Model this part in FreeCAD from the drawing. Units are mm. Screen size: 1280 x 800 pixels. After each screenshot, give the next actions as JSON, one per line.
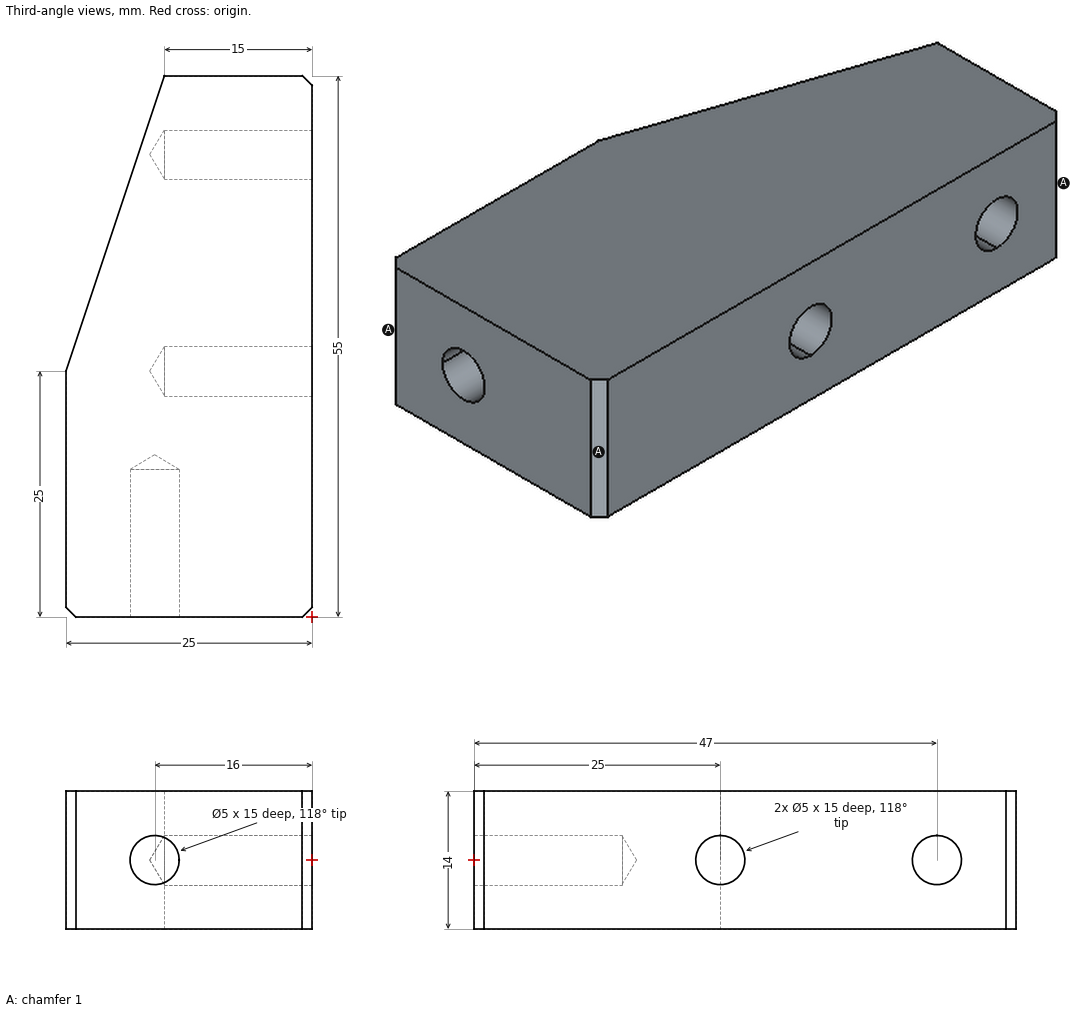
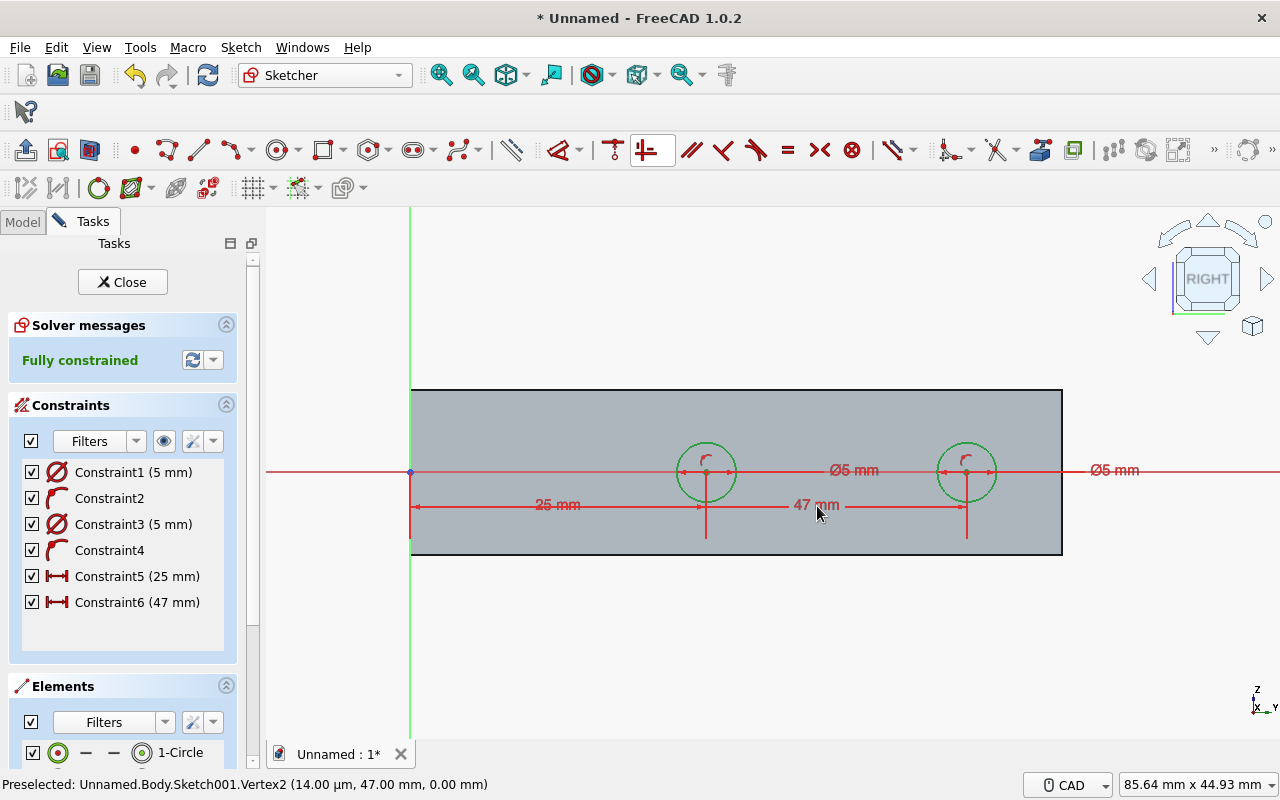
{"action": "left_click", "coordinate": [123, 282]}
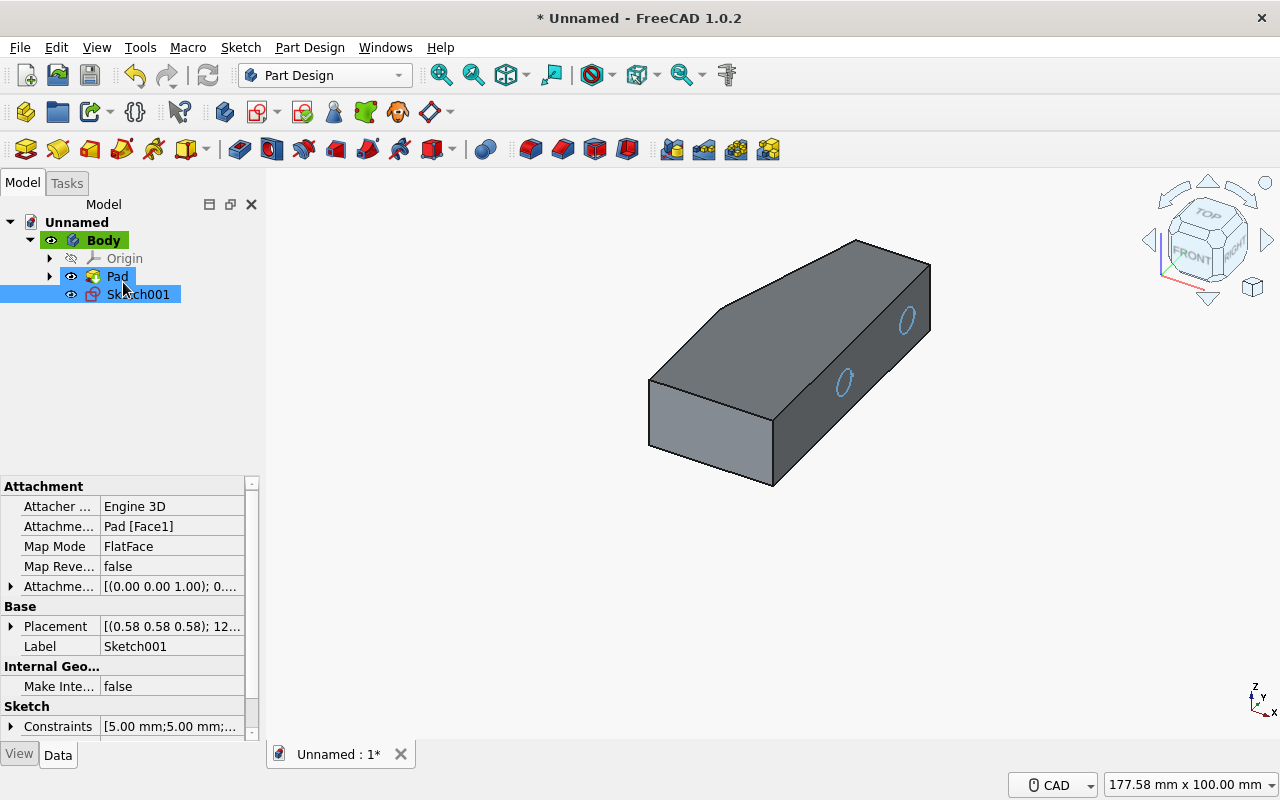
{"action": "left_click", "coordinate": [272, 150]}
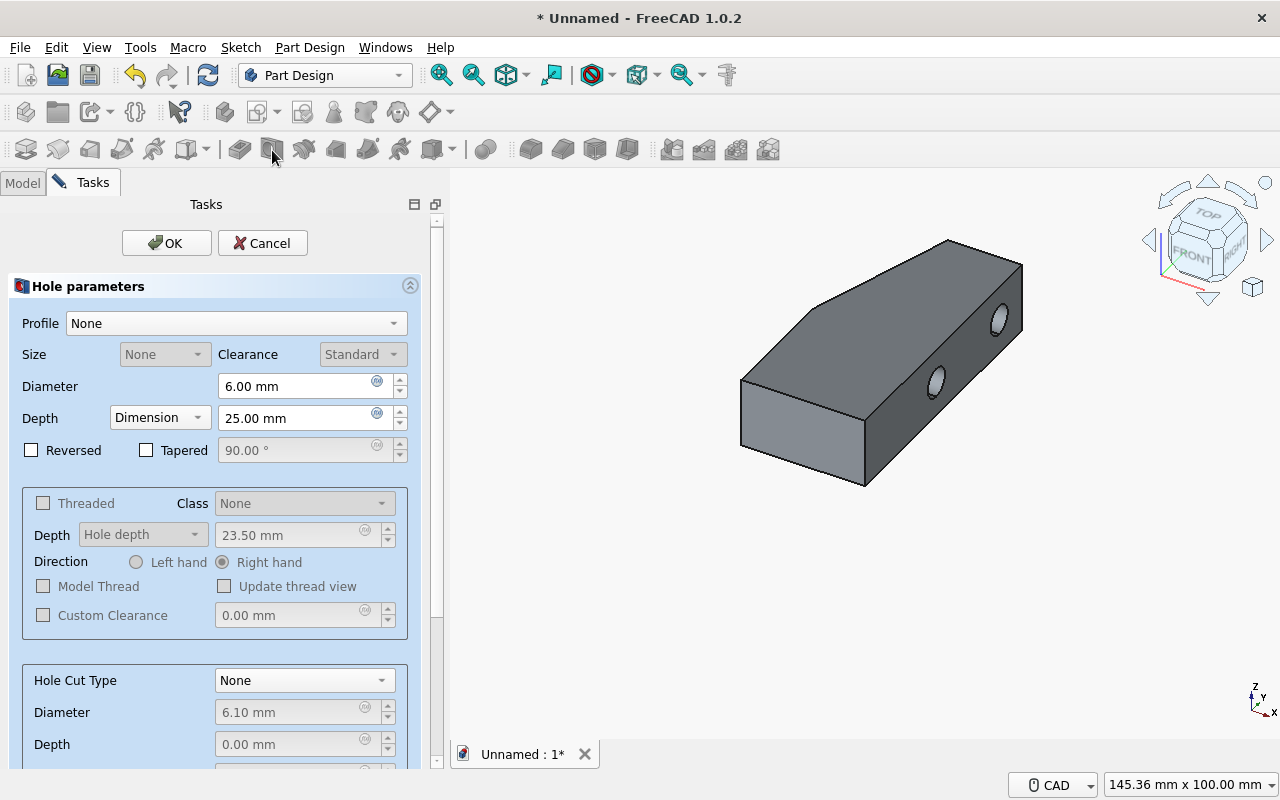
{"action": "triple_click", "coordinate": [305, 386]}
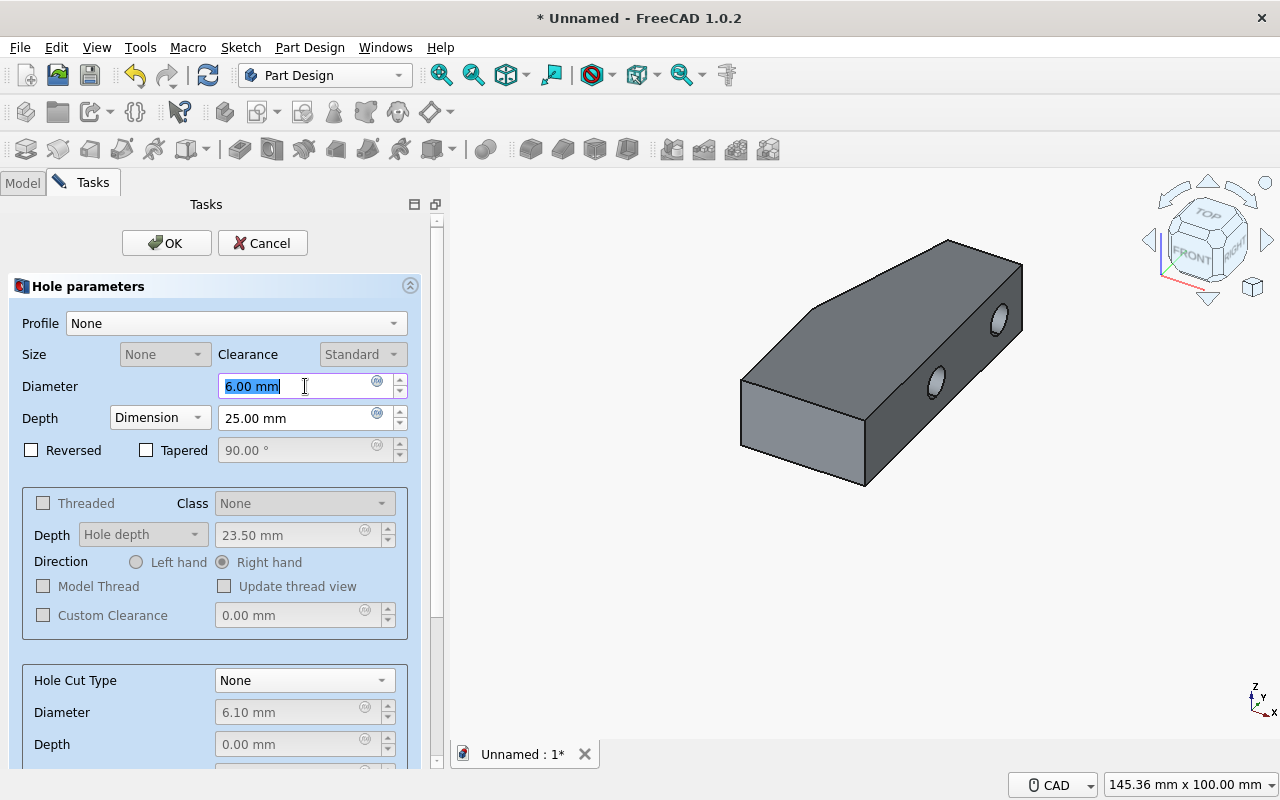
{"action": "type", "text": "5"}
{"action": "key", "text": "Tab"}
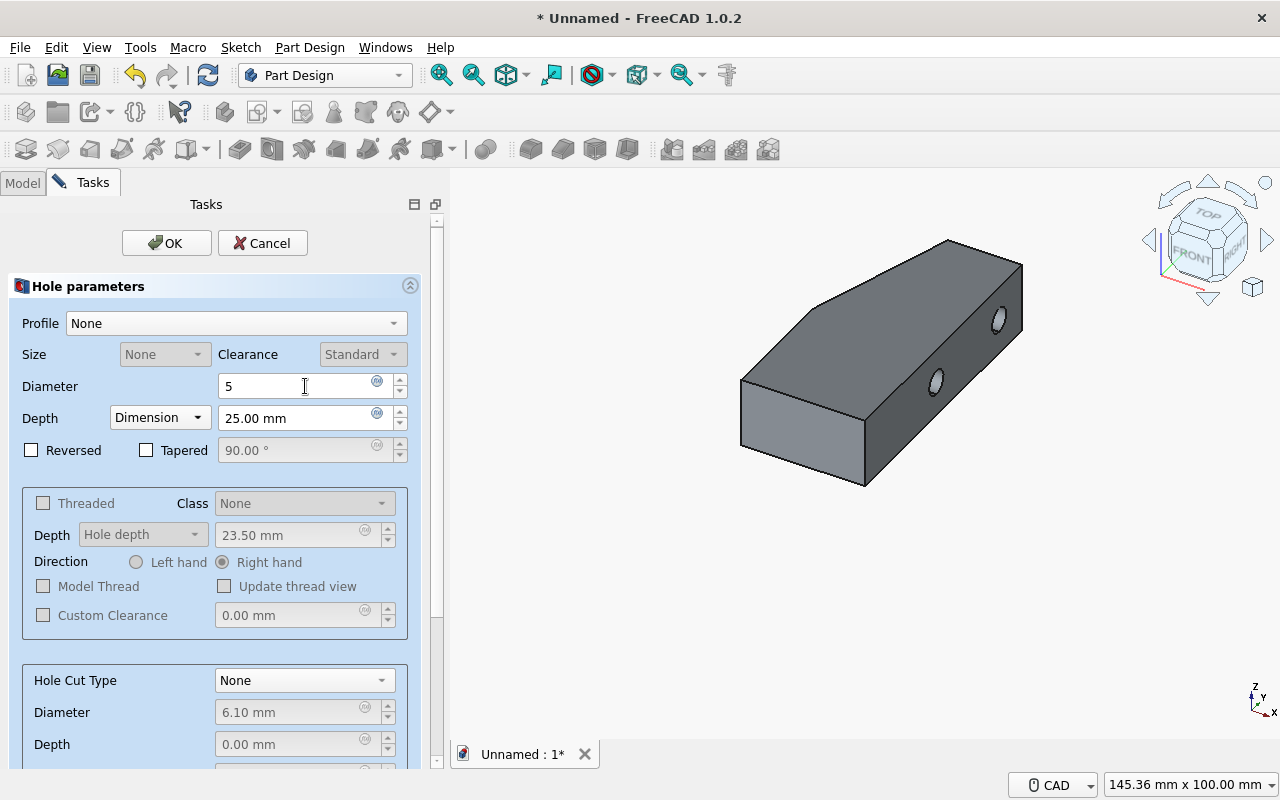
{"action": "triple_click", "coordinate": [305, 418]}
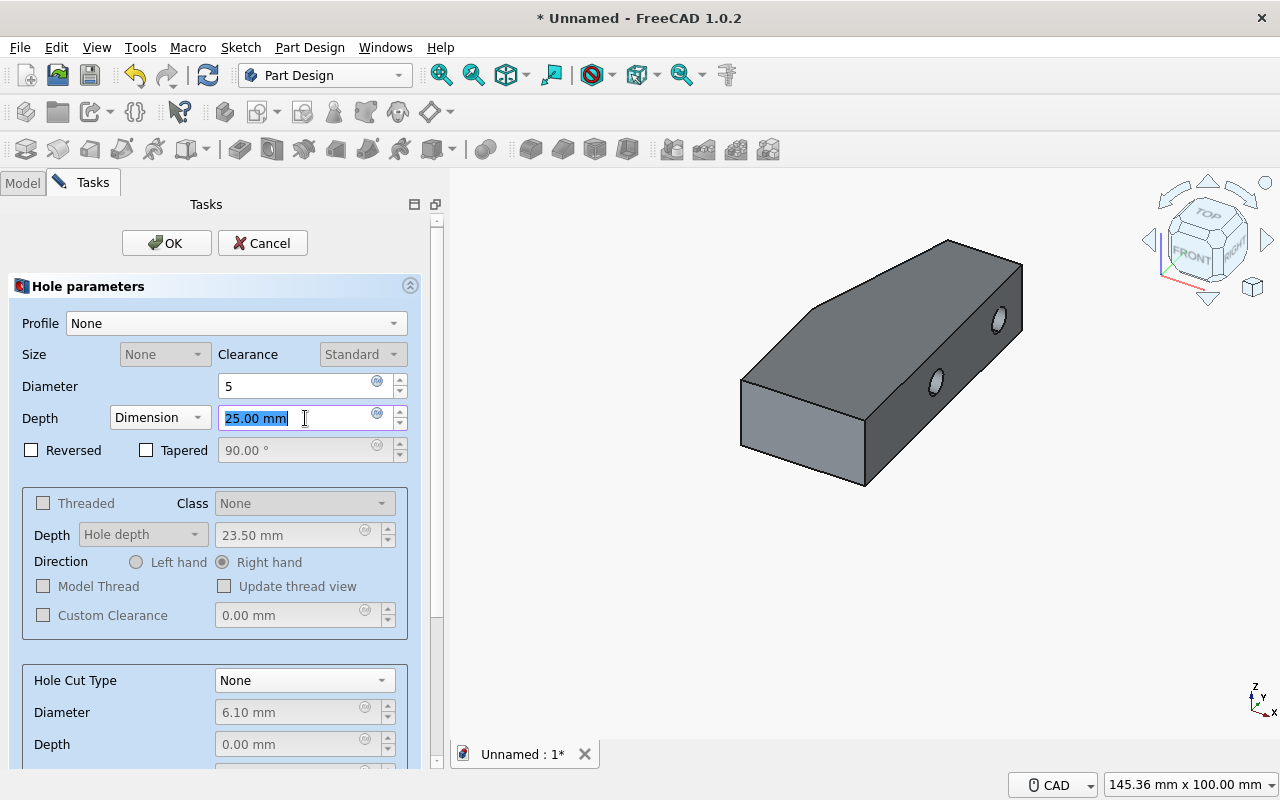
{"action": "type", "text": "15"}
{"action": "key", "text": "Tab"}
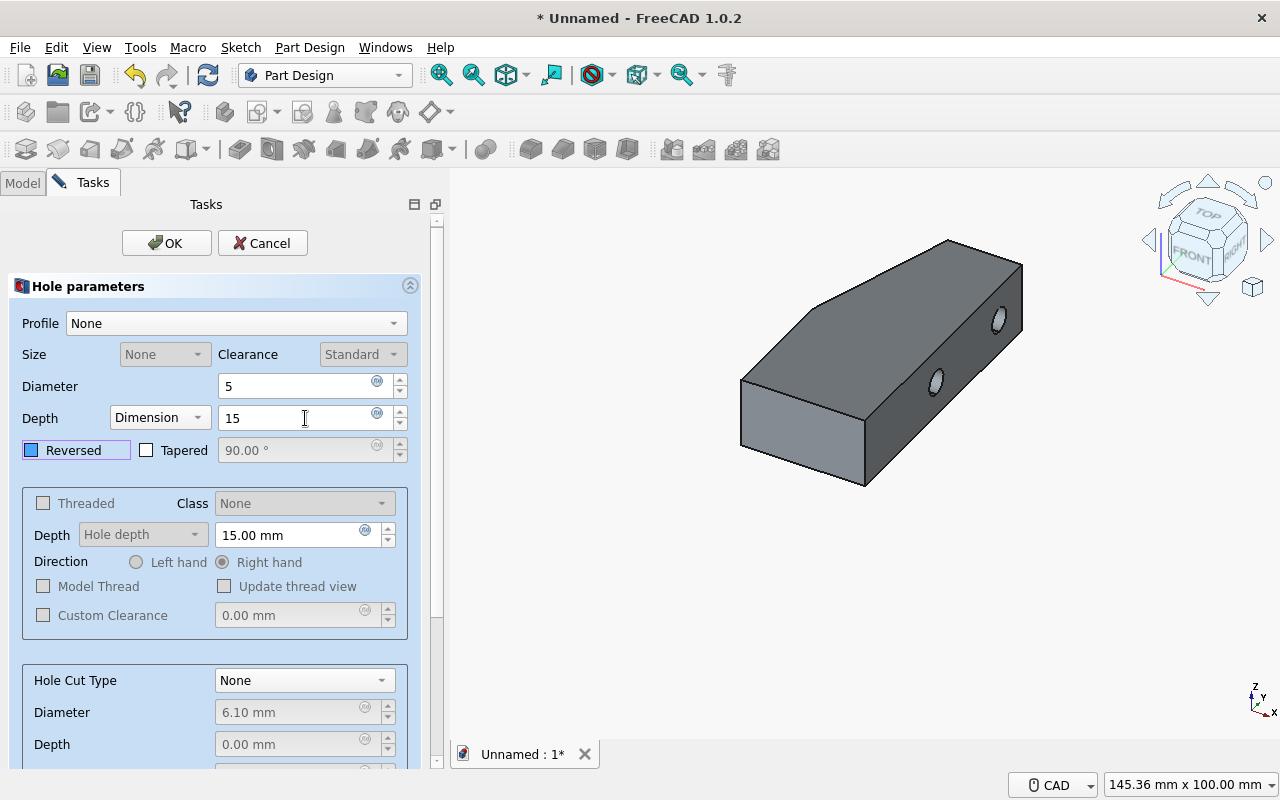
{"action": "left_click", "coordinate": [167, 243]}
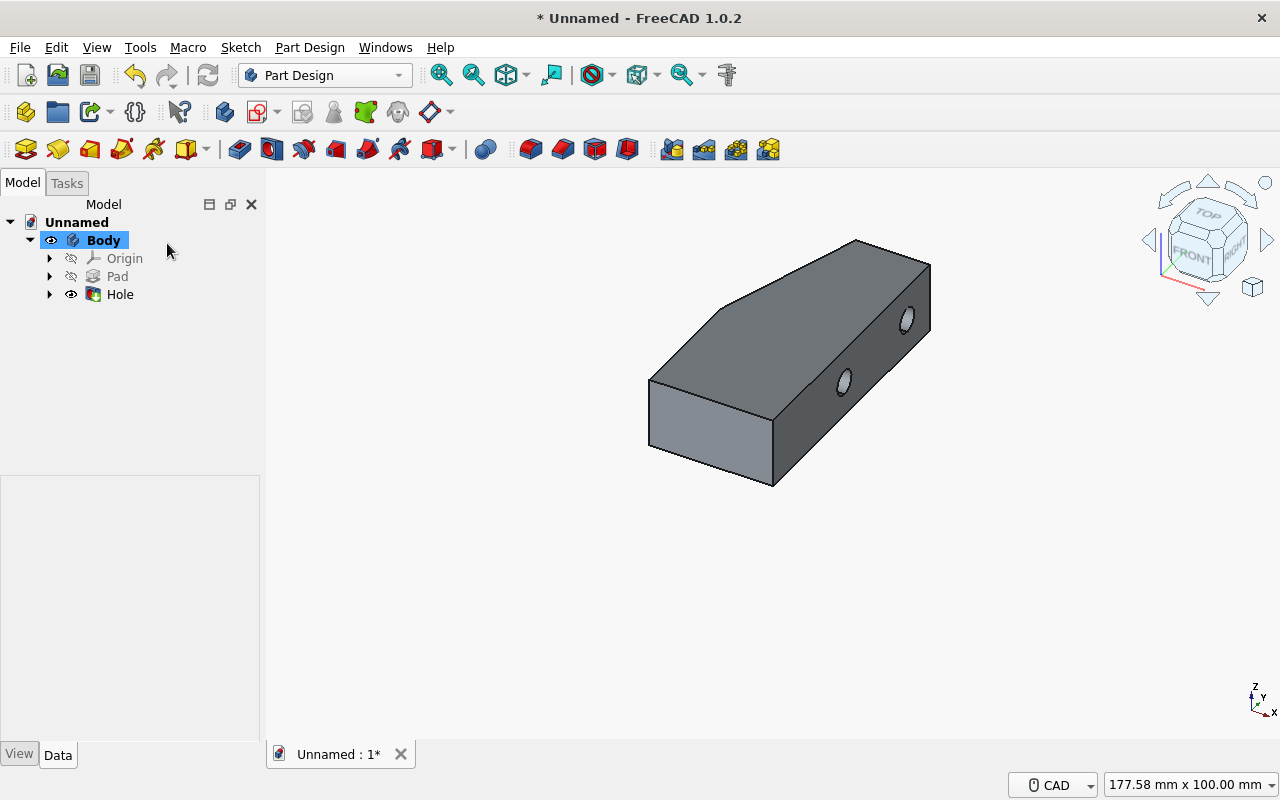
{"action": "left_click", "coordinate": [258, 112]}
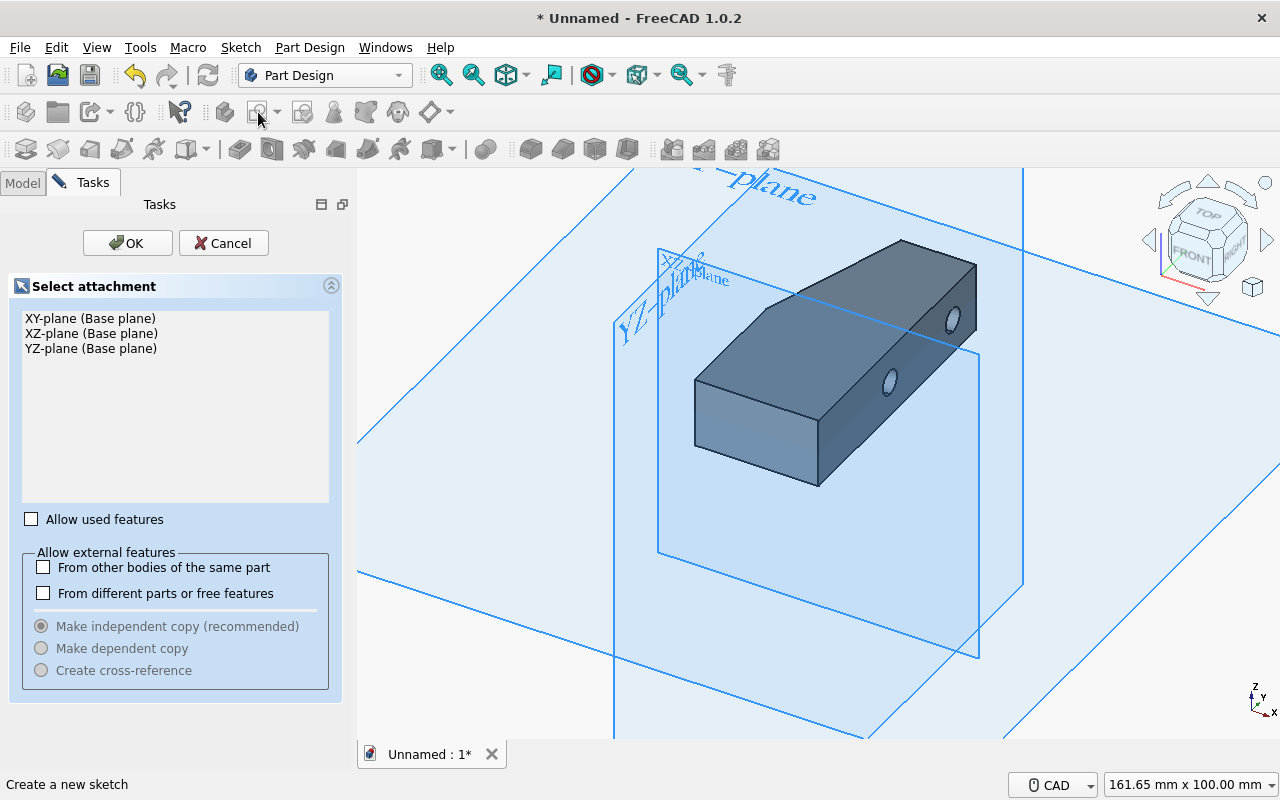
{"action": "left_click", "coordinate": [82, 334]}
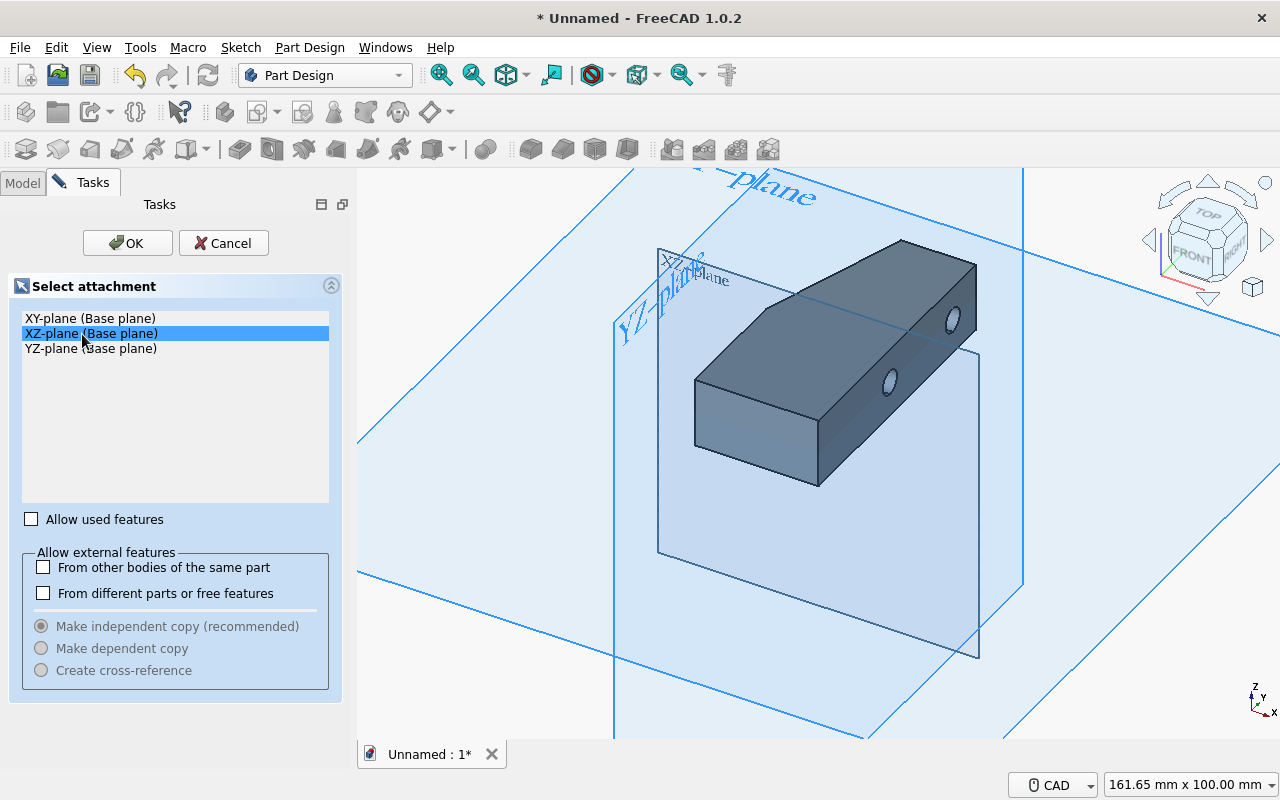
{"action": "left_click", "coordinate": [128, 243]}